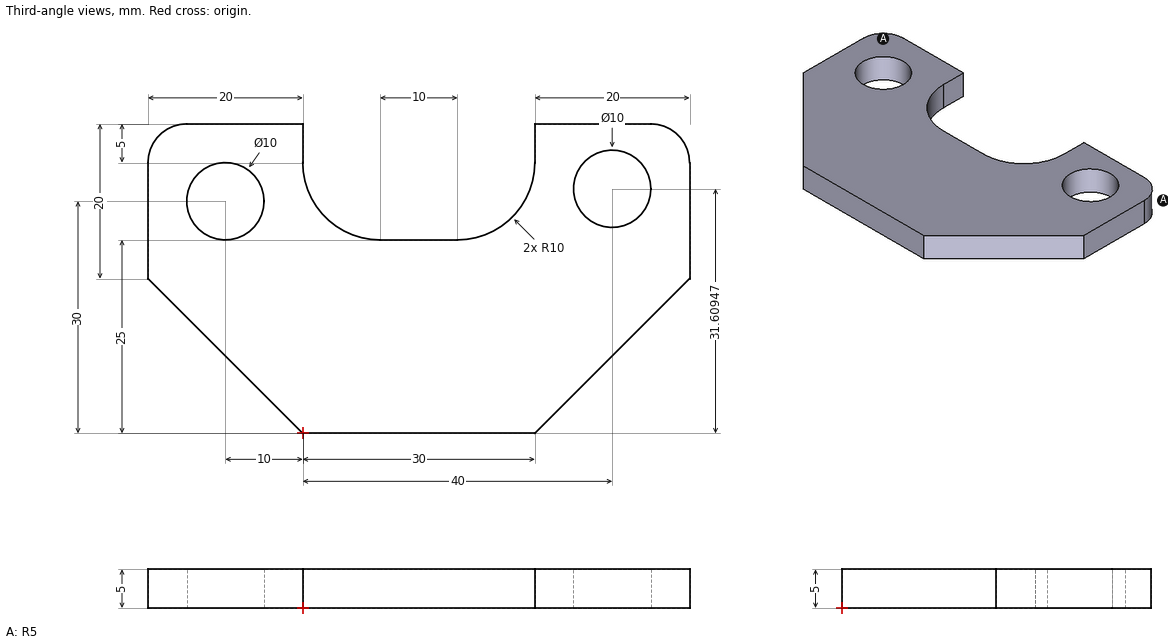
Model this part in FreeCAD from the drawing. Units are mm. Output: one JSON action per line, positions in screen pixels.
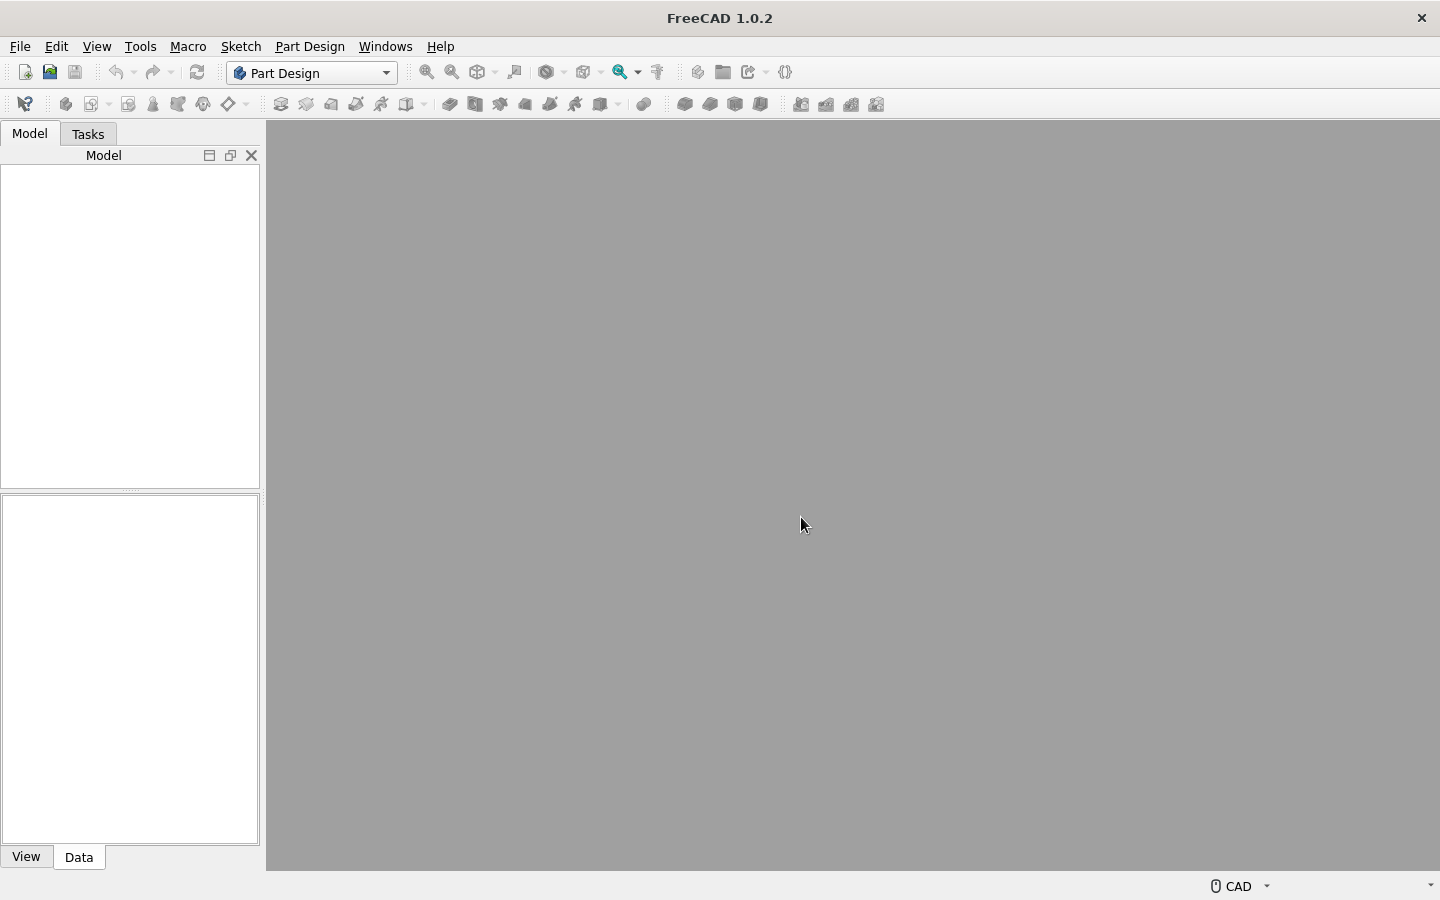
{"action": "left_click", "coordinate": [25, 72]}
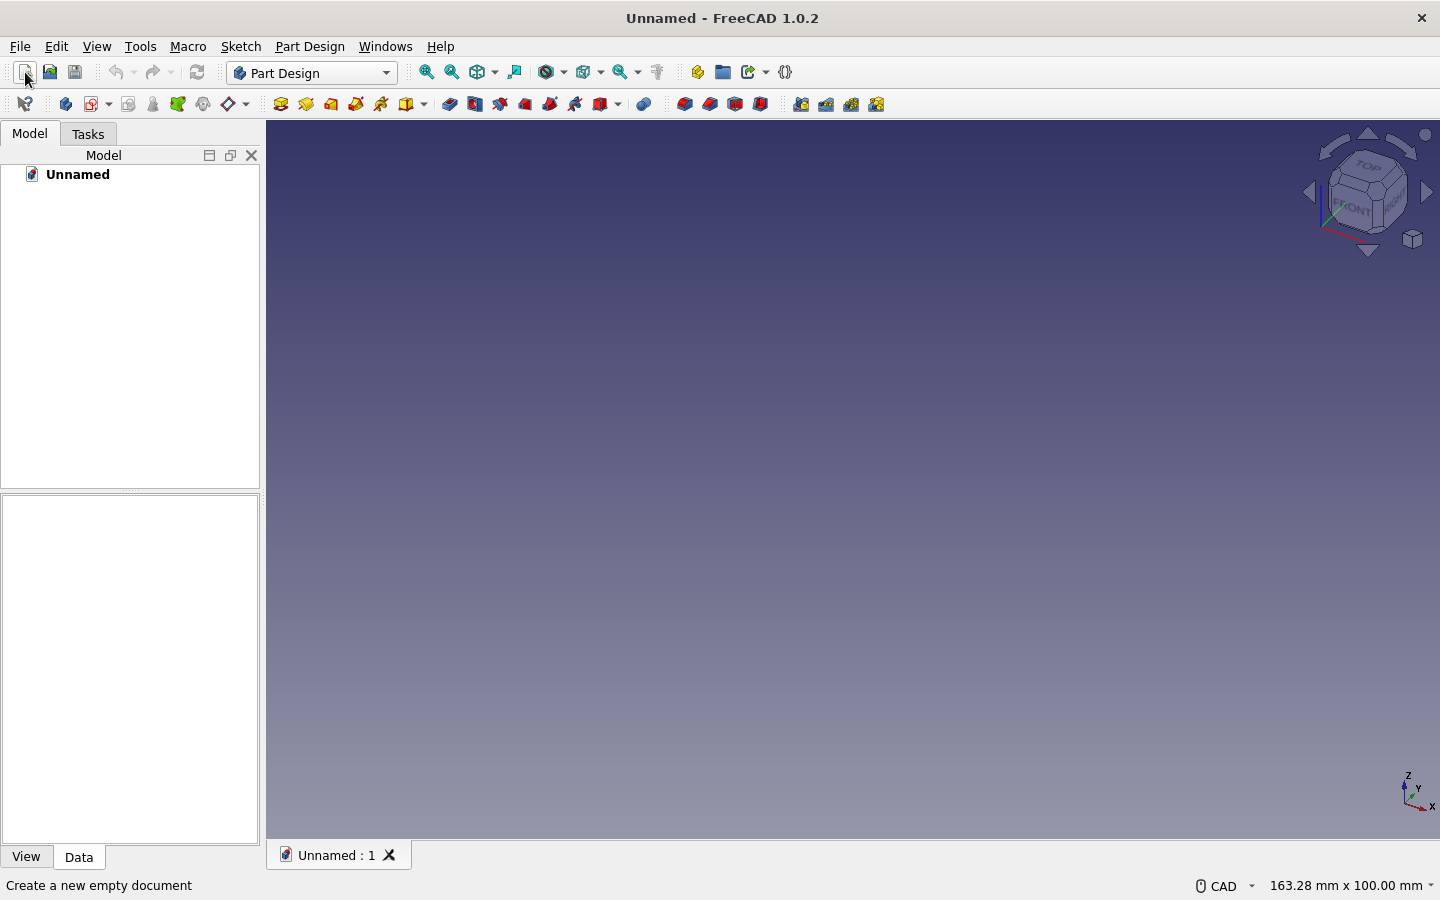
{"action": "left_click", "coordinate": [90, 104]}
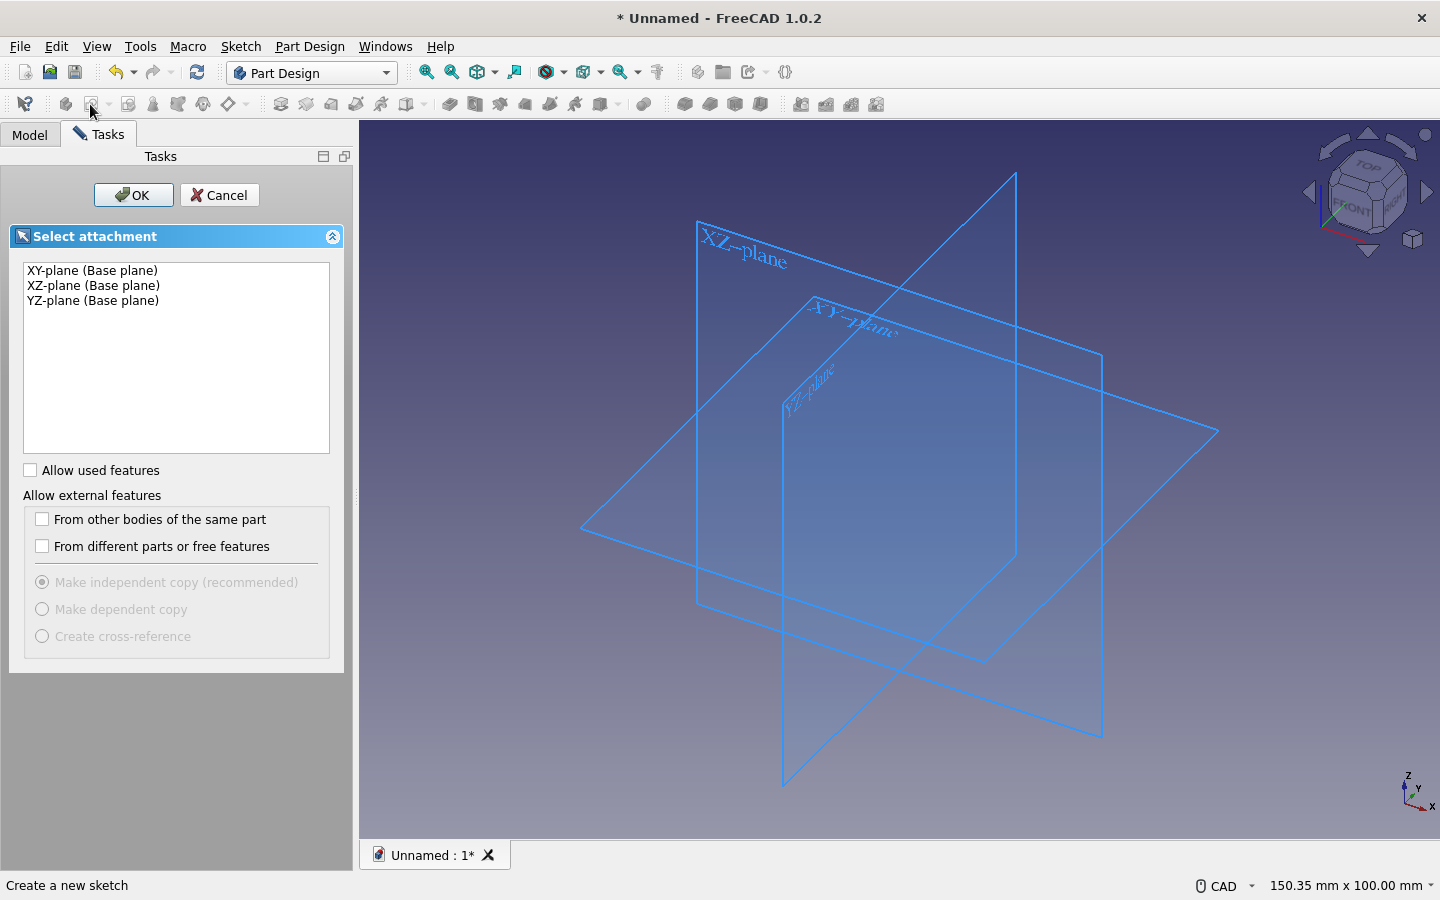
{"action": "left_click", "coordinate": [84, 270]}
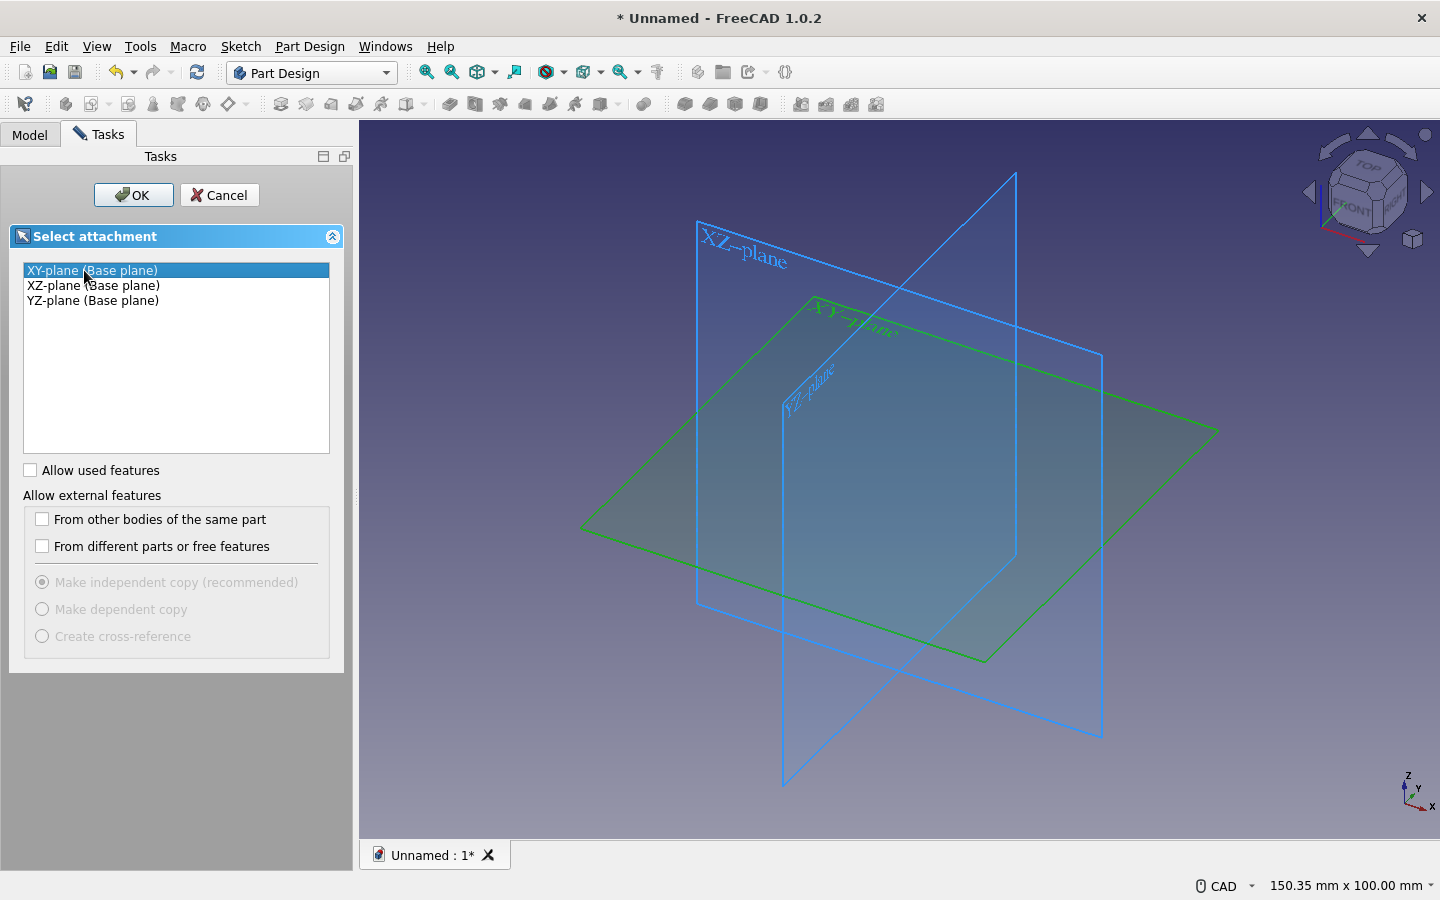
{"action": "left_click", "coordinate": [134, 195]}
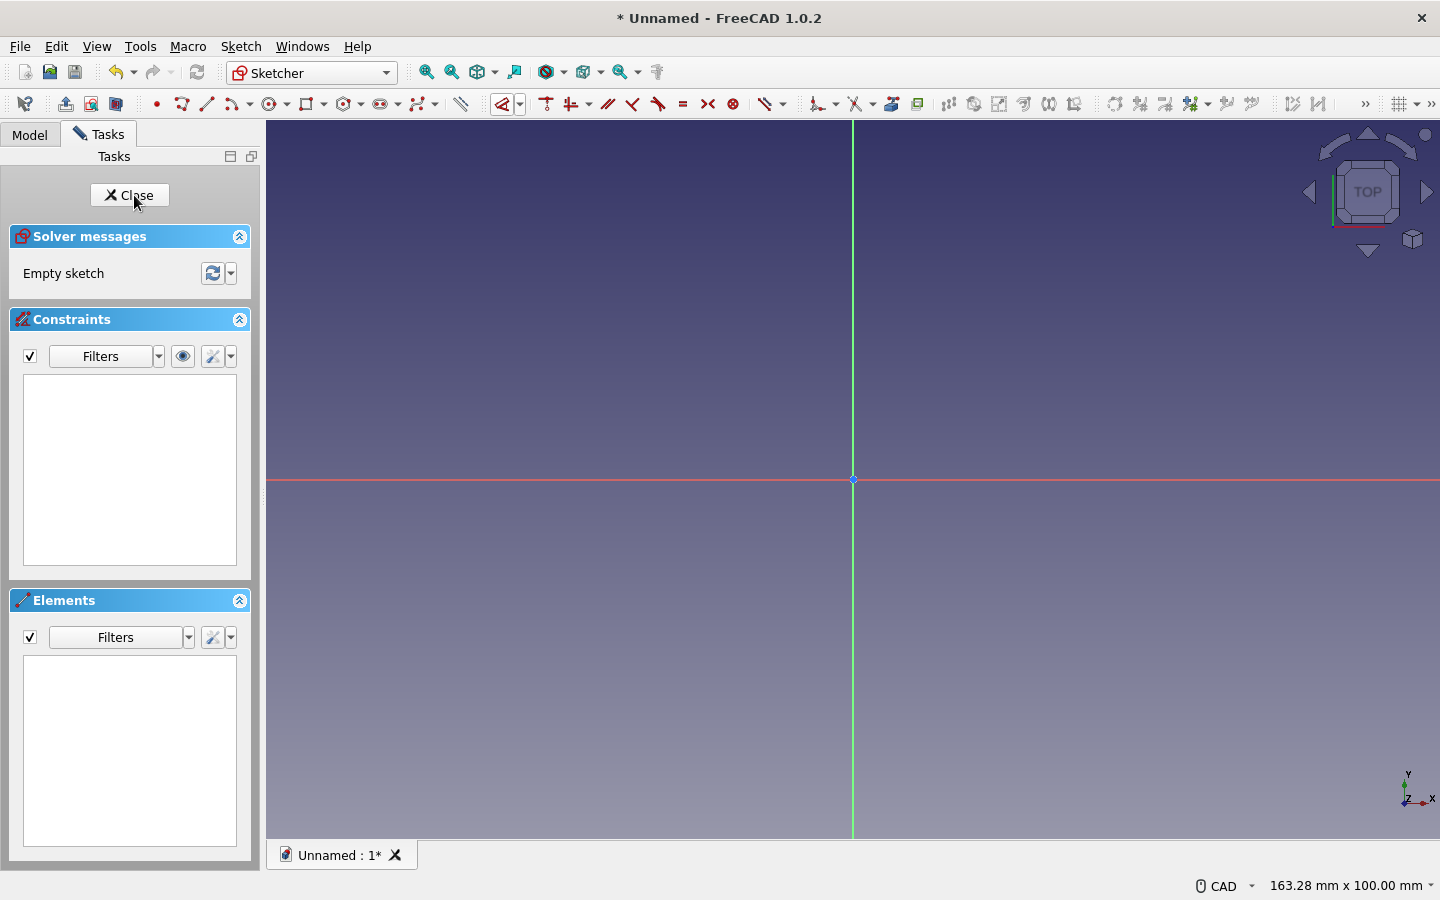
{"action": "scroll", "coordinate": [1275, 148], "scroll_direction": "up", "scroll_amount": 2}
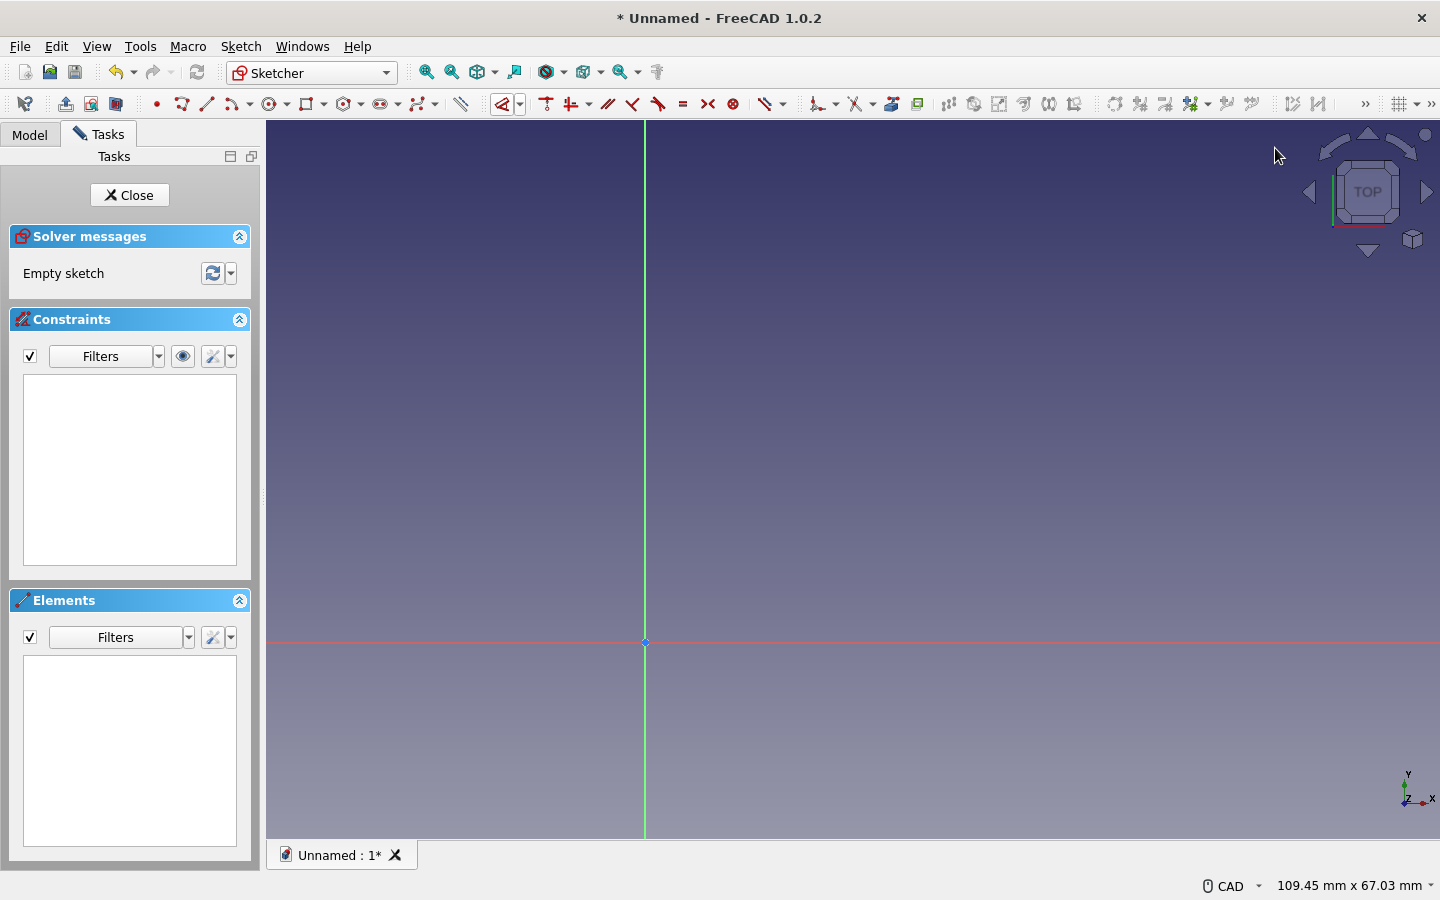
{"action": "left_click", "coordinate": [207, 104]}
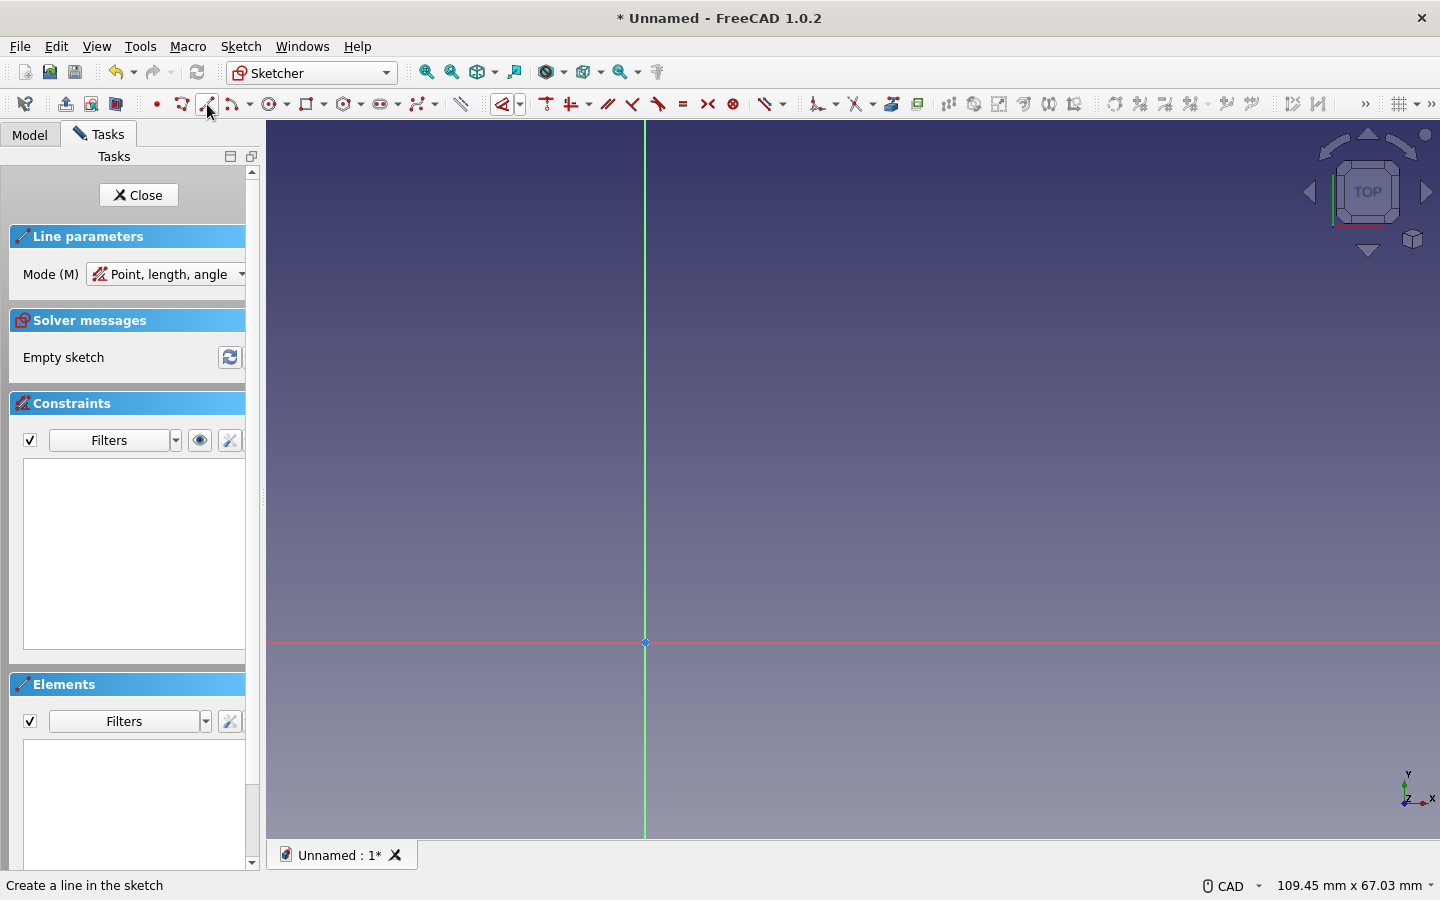
{"action": "left_click", "coordinate": [860, 374]}
{"action": "left_click", "coordinate": [752, 374]}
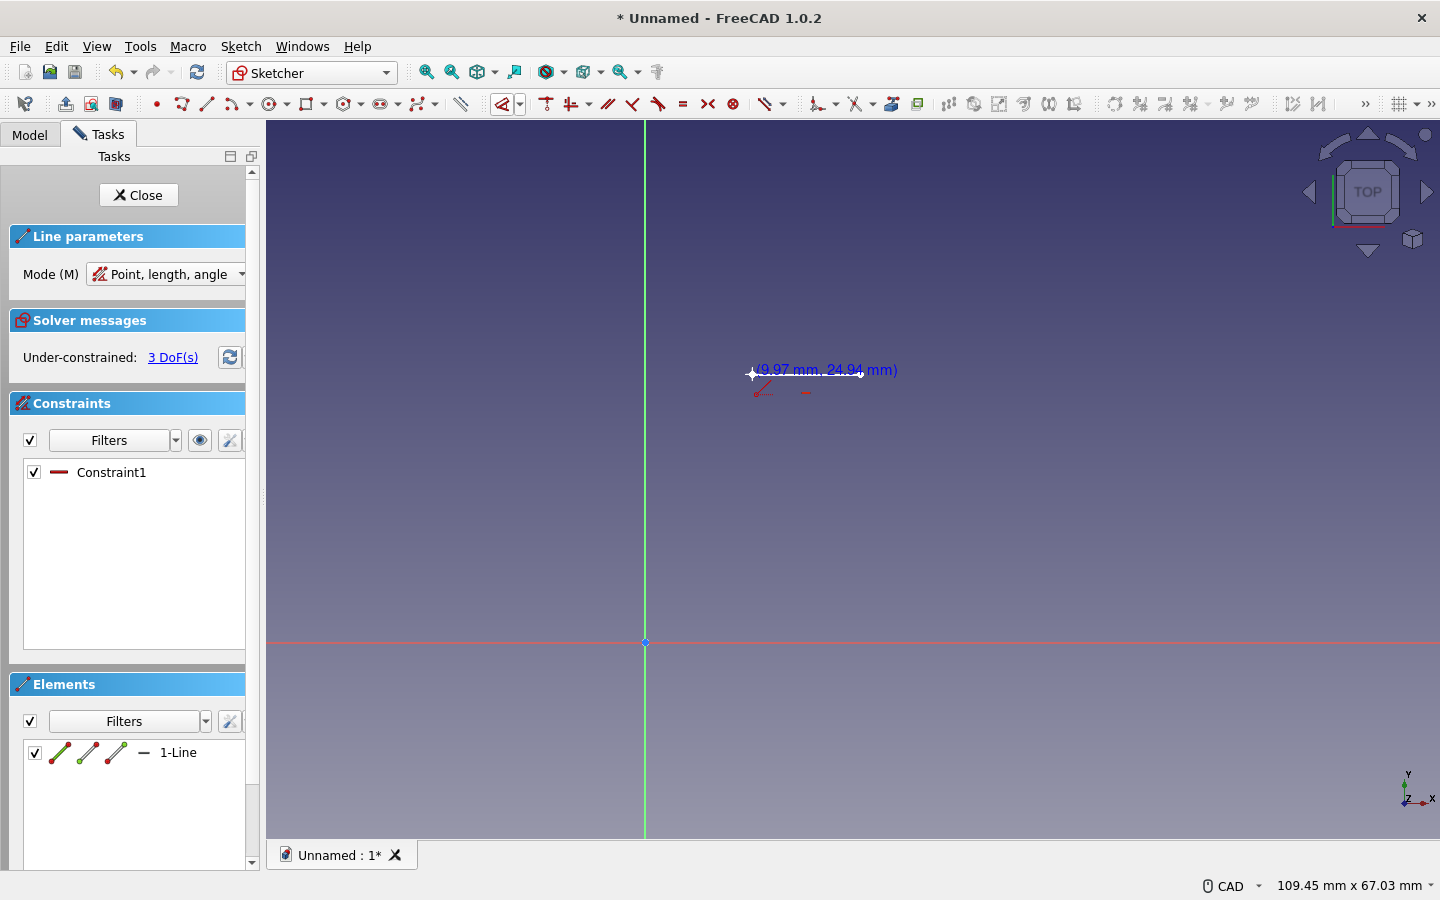
{"action": "left_click", "coordinate": [182, 104]}